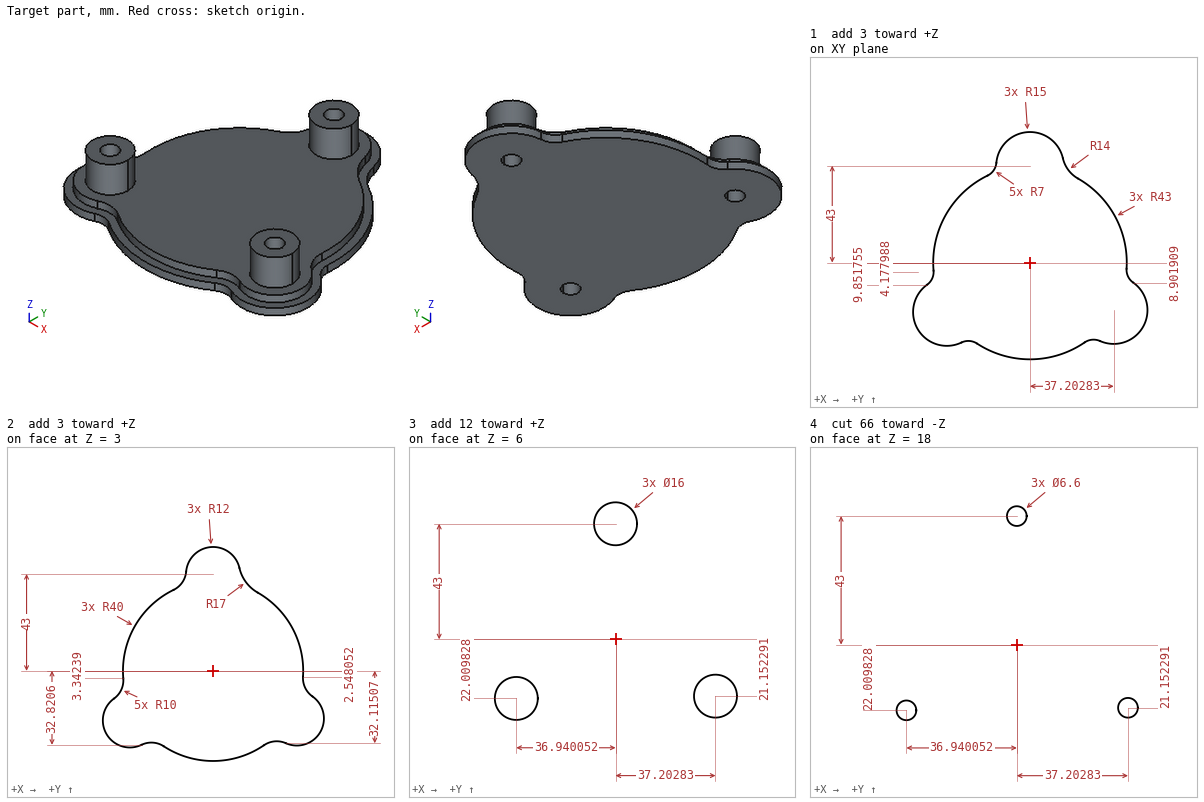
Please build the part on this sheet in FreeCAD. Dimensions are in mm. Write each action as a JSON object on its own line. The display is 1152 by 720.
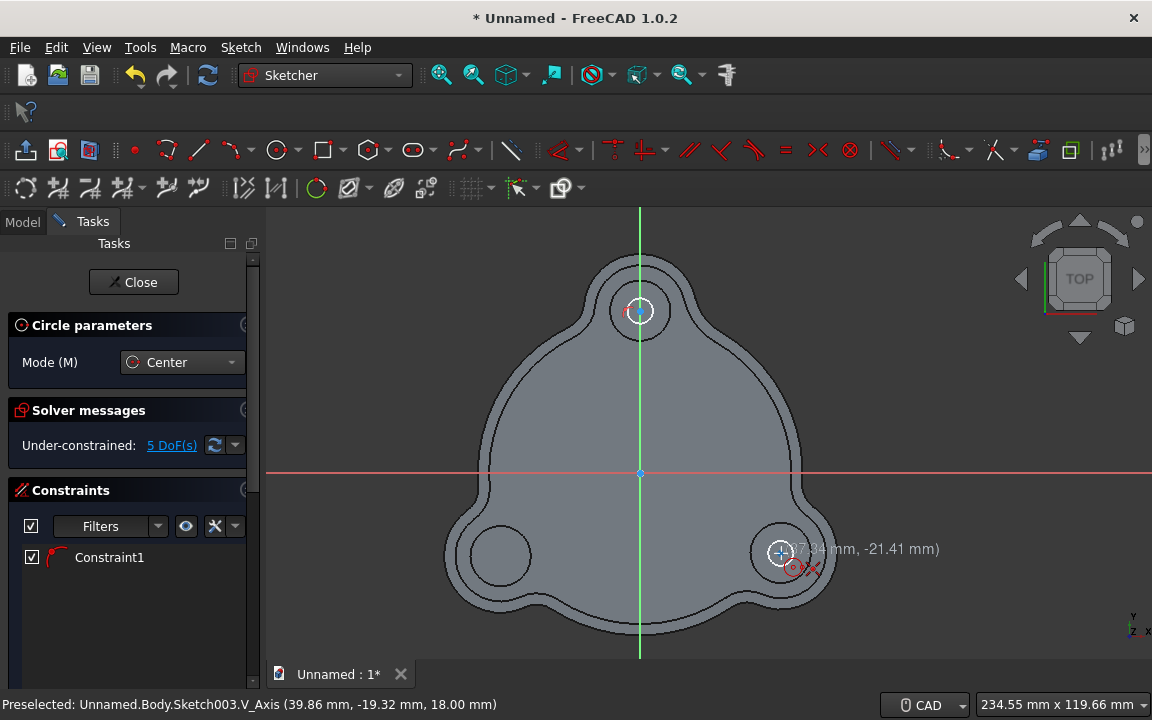
{"action": "scroll", "coordinate": [501, 556], "scroll_direction": "up", "scroll_amount": 3}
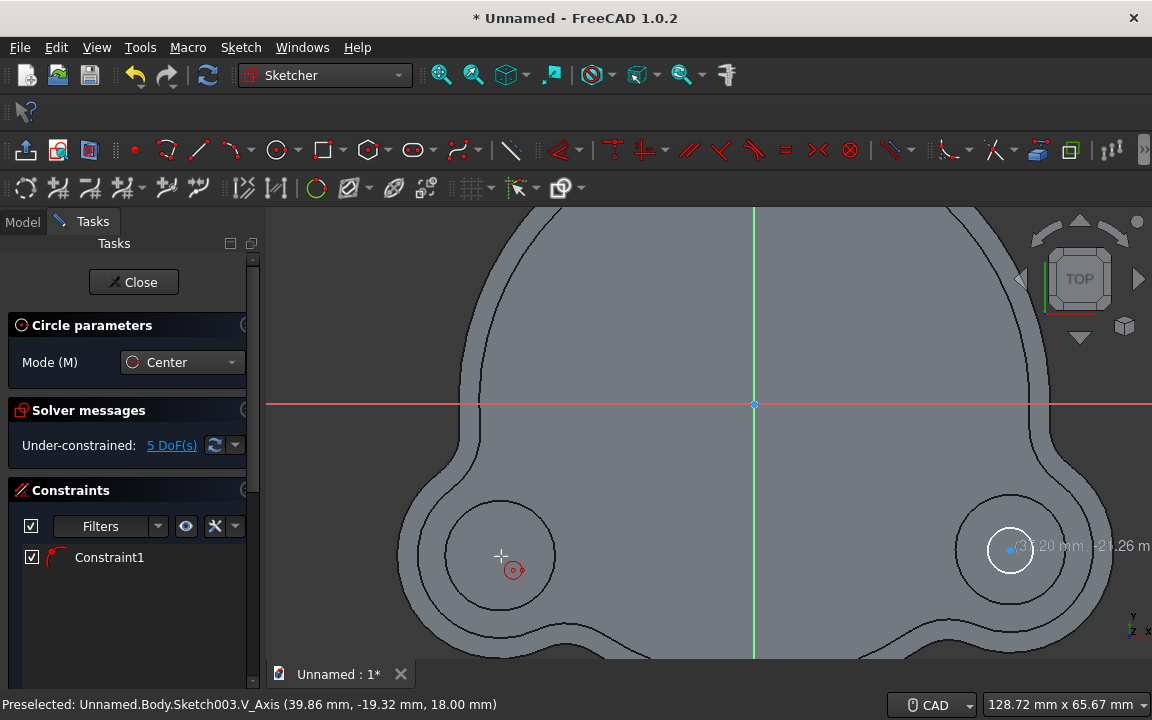
{"action": "left_click", "coordinate": [500, 556]}
{"action": "left_click", "coordinate": [516, 540]}
{"action": "key", "text": "Escape"}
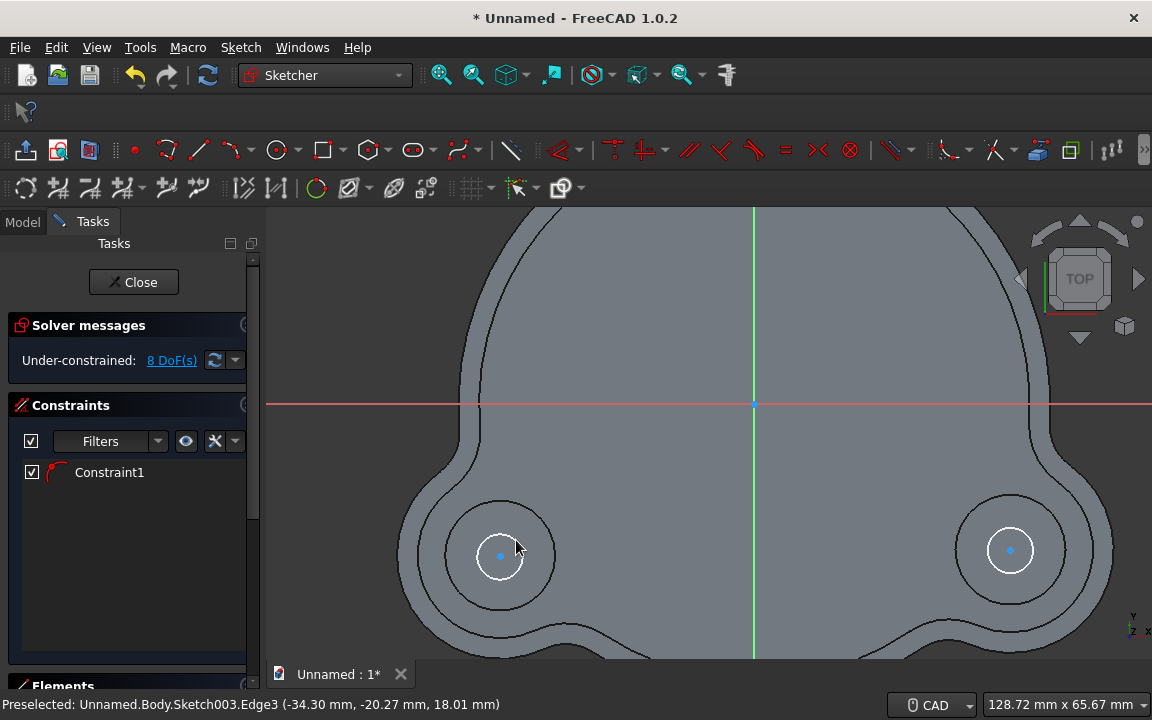
{"action": "scroll", "coordinate": [501, 556], "scroll_direction": "down", "scroll_amount": 3}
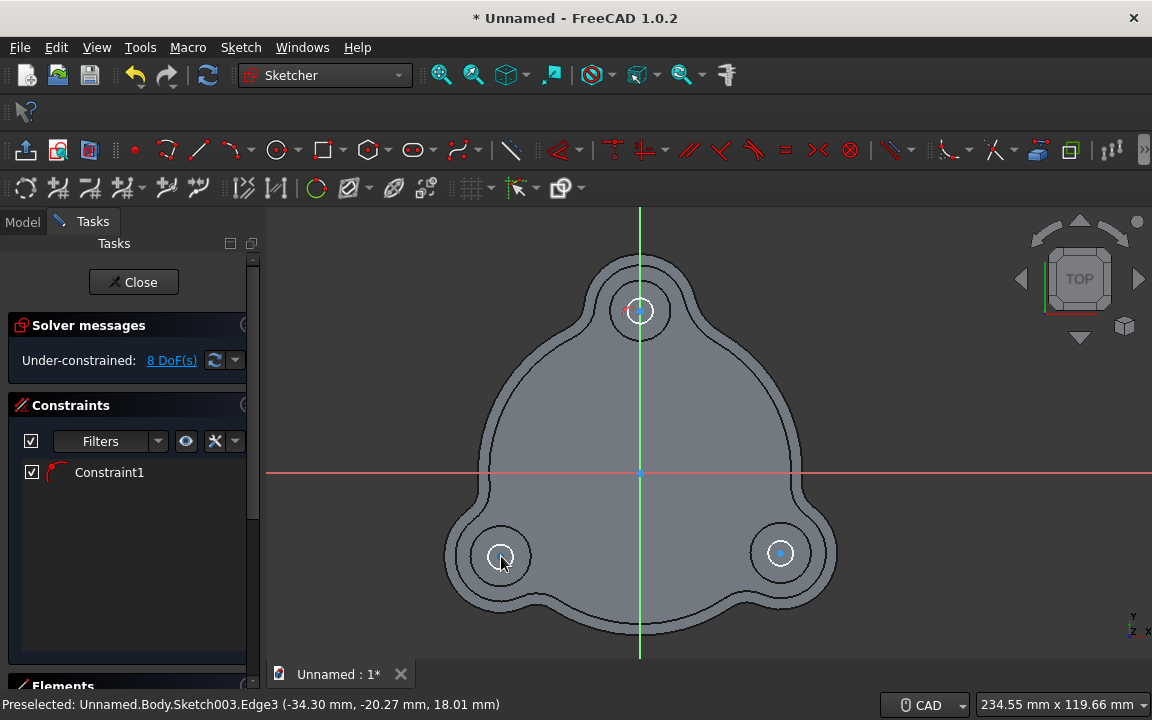
{"action": "scroll", "coordinate": [649, 302], "scroll_direction": "up", "scroll_amount": 3}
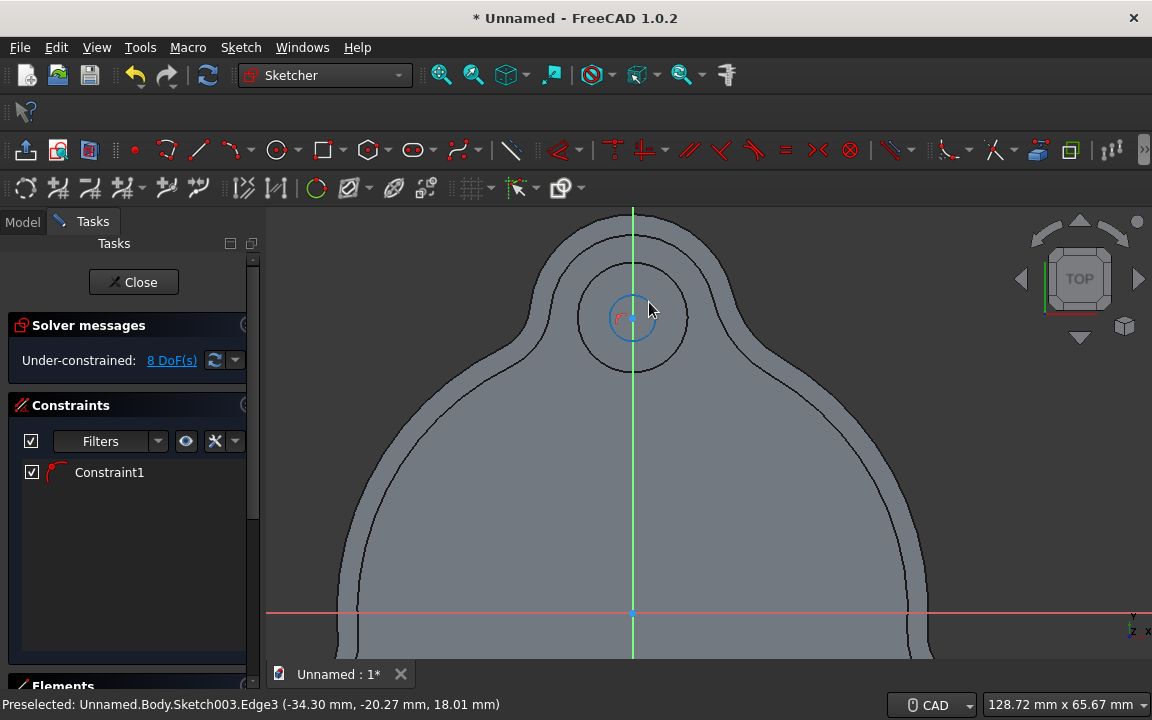
{"action": "left_click", "coordinate": [649, 302]}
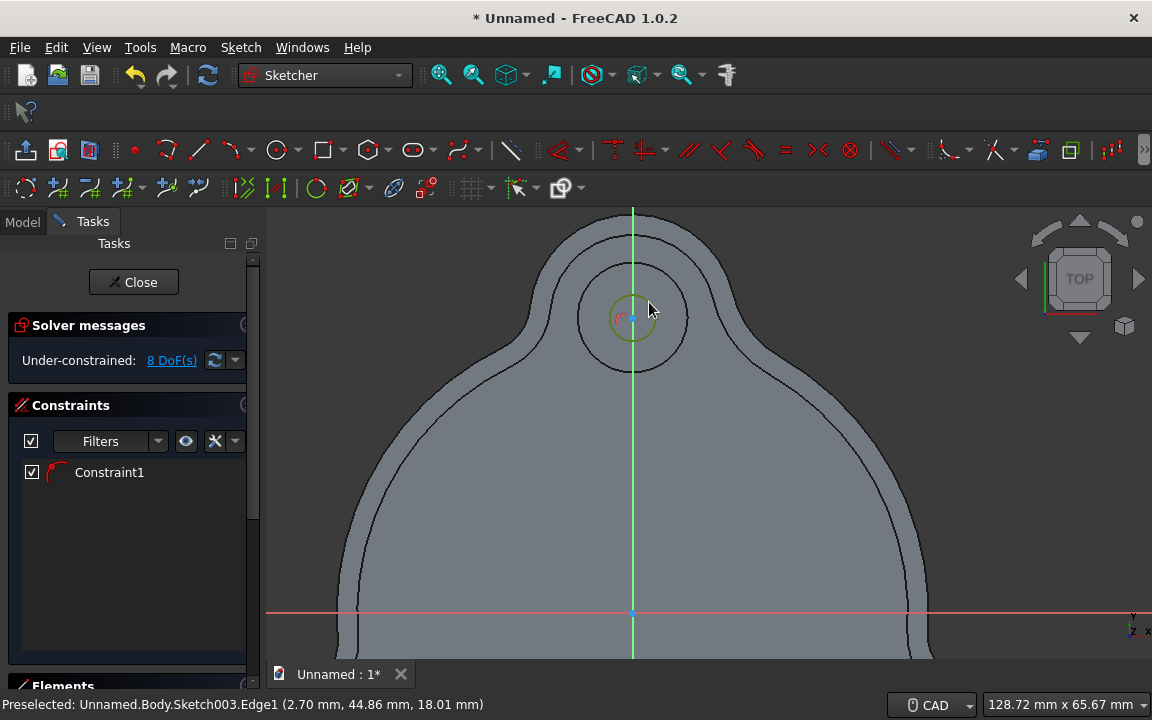
{"action": "scroll", "coordinate": [649, 301], "scroll_direction": "down", "scroll_amount": 3}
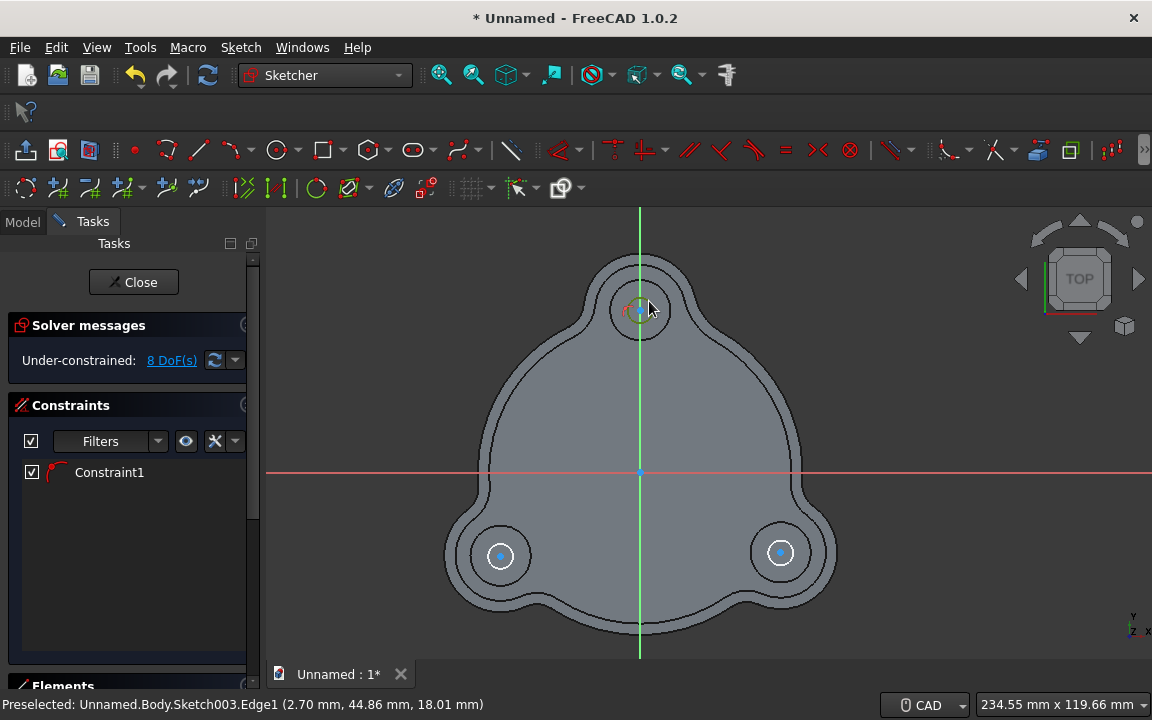
{"action": "left_click", "coordinate": [789, 544]}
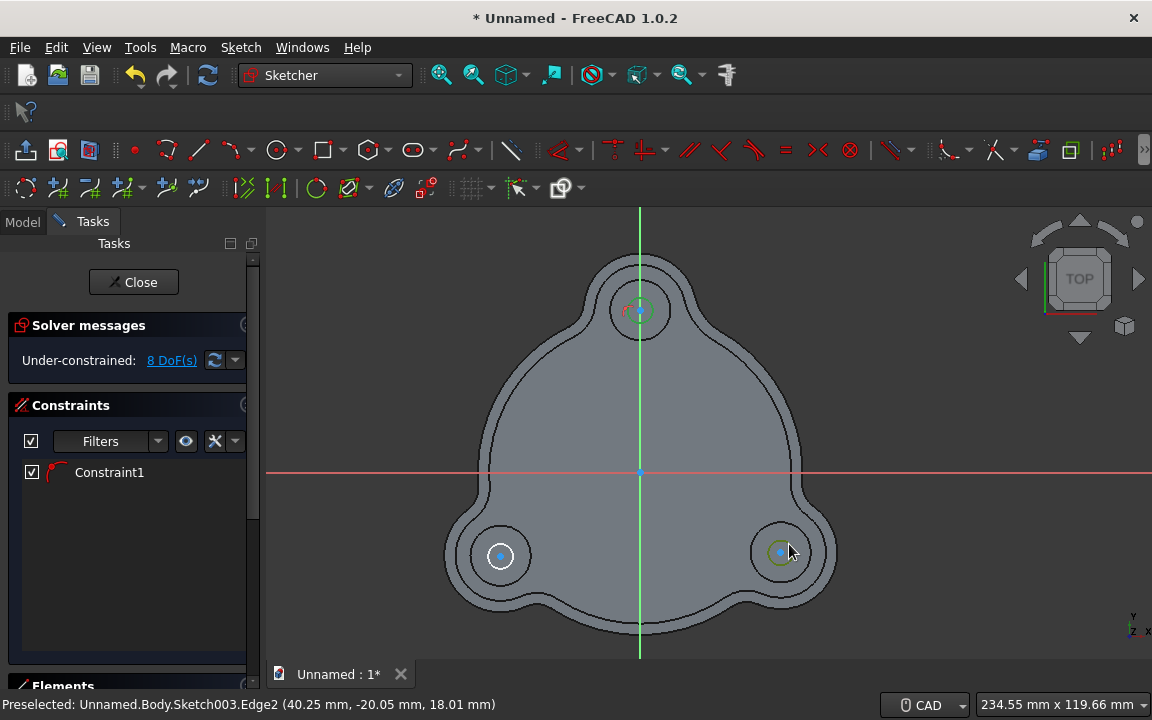
{"action": "left_click", "coordinate": [509, 548]}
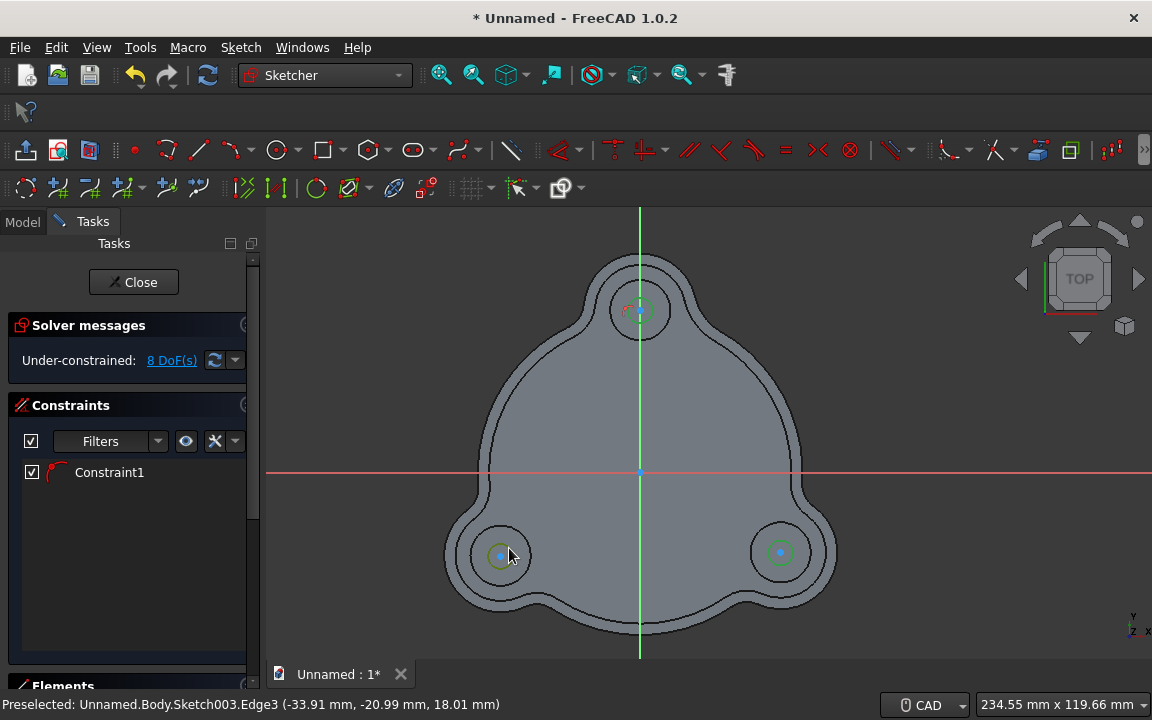
{"action": "left_click", "coordinate": [786, 150]}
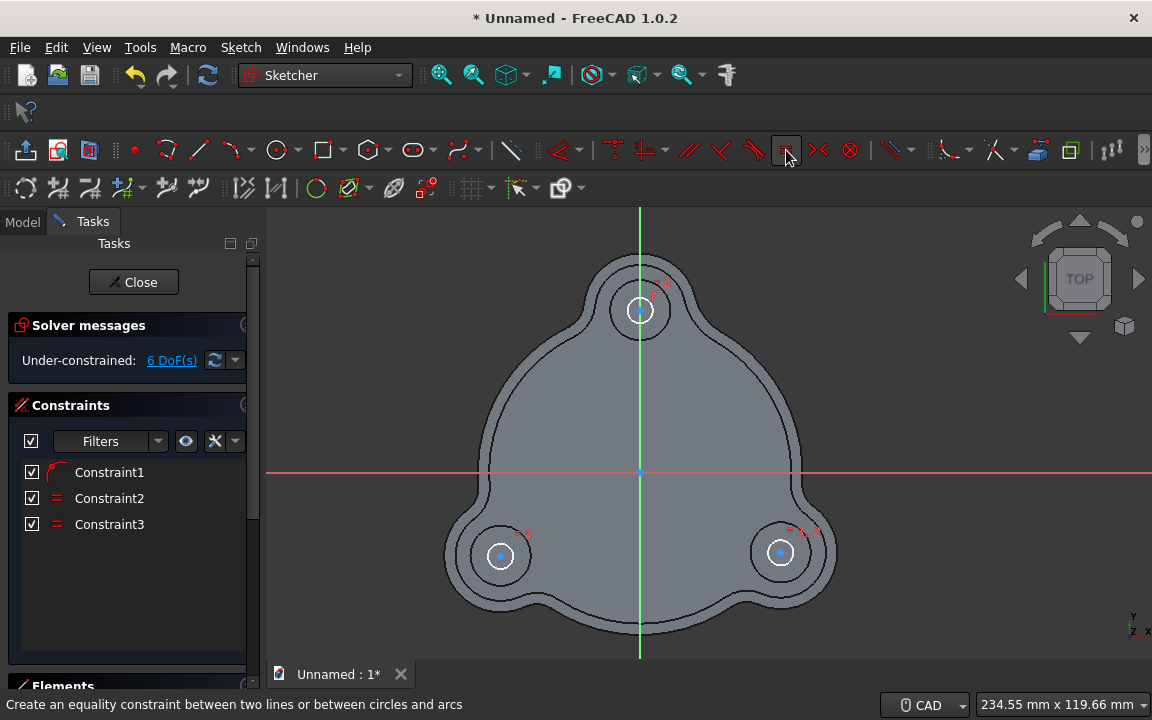
{"action": "left_click", "coordinate": [558, 150]}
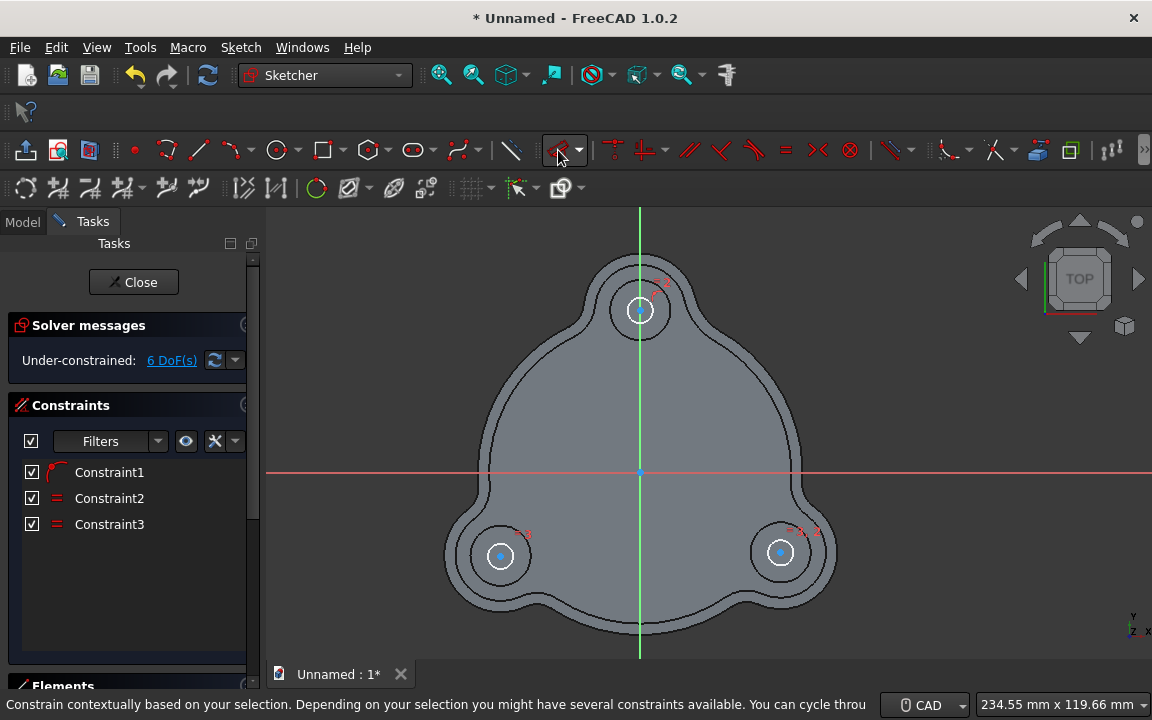
{"action": "scroll", "coordinate": [641, 298], "scroll_direction": "up", "scroll_amount": 3}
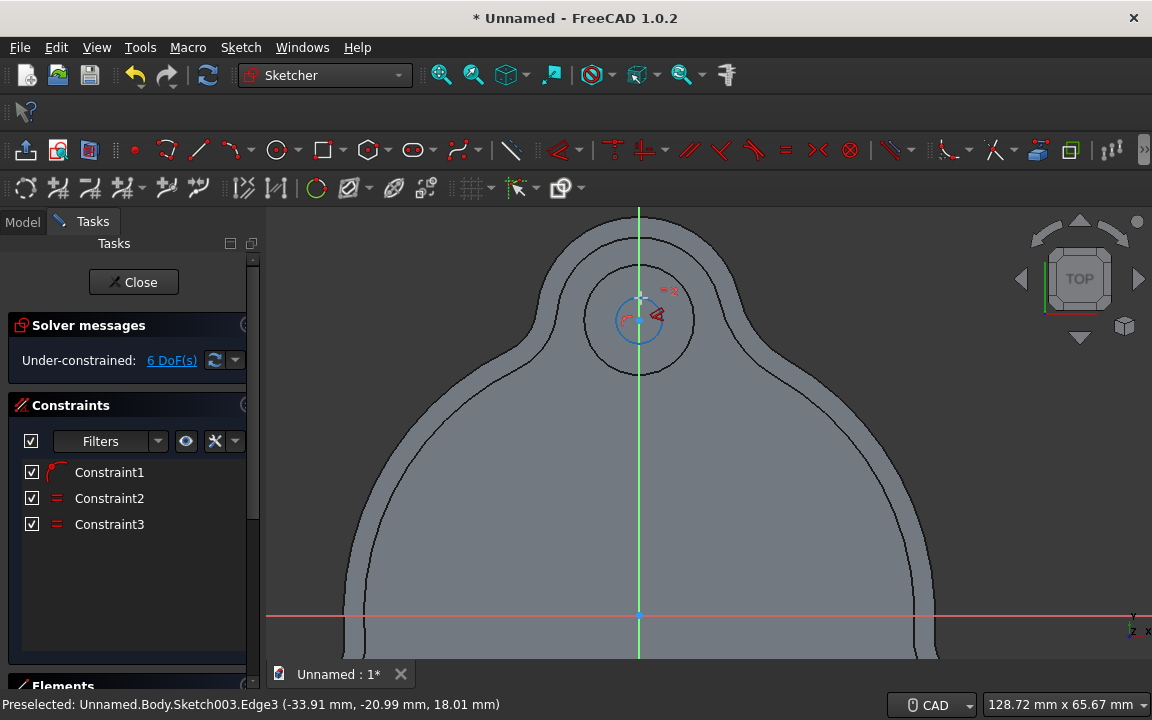
{"action": "left_click", "coordinate": [640, 298]}
{"action": "left_click", "coordinate": [667, 274]}